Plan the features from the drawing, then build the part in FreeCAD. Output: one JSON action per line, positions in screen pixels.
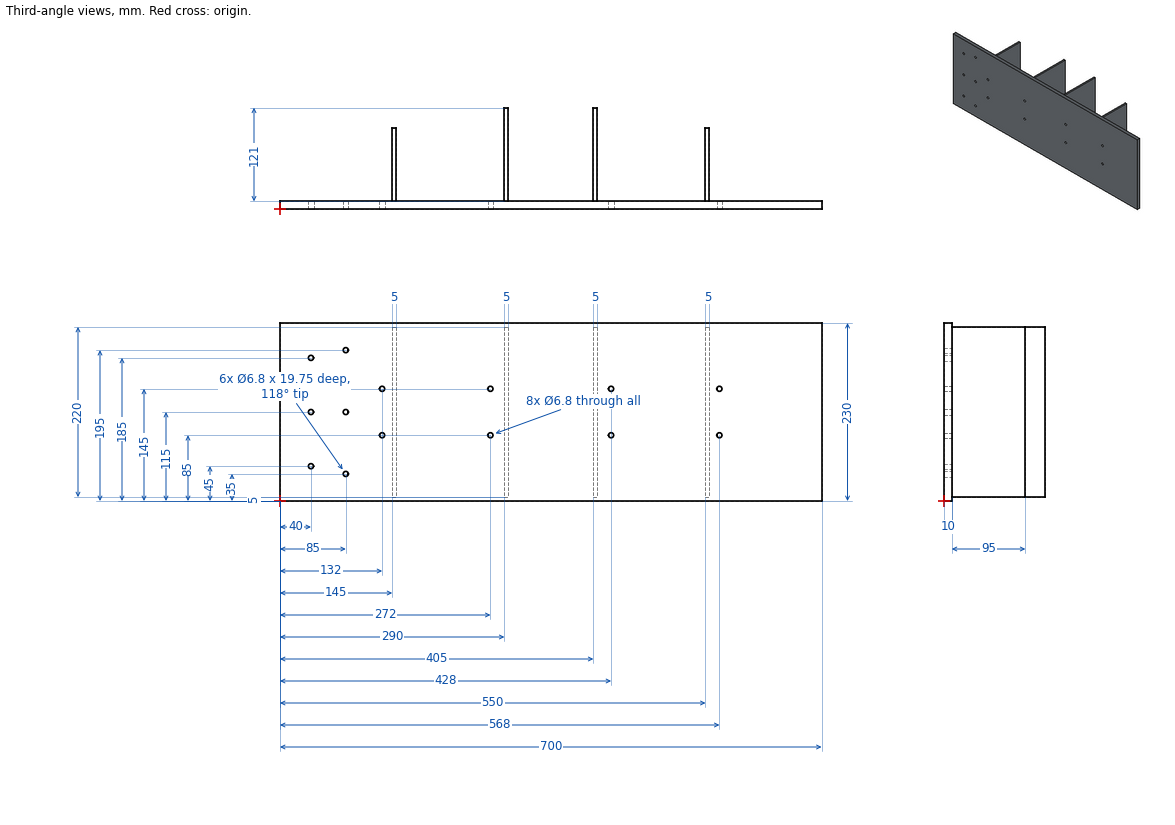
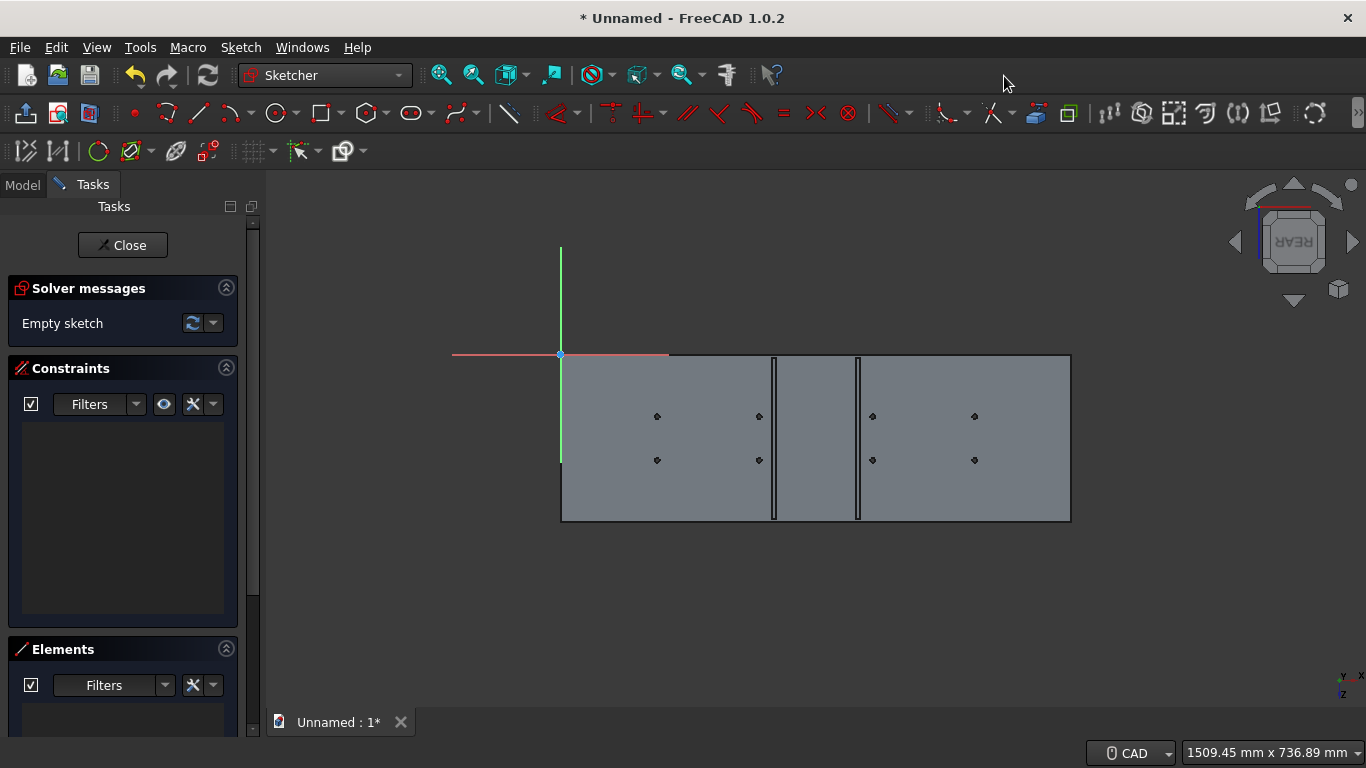
{"action": "scroll", "coordinate": [795, 433], "scroll_direction": "up", "scroll_amount": 2}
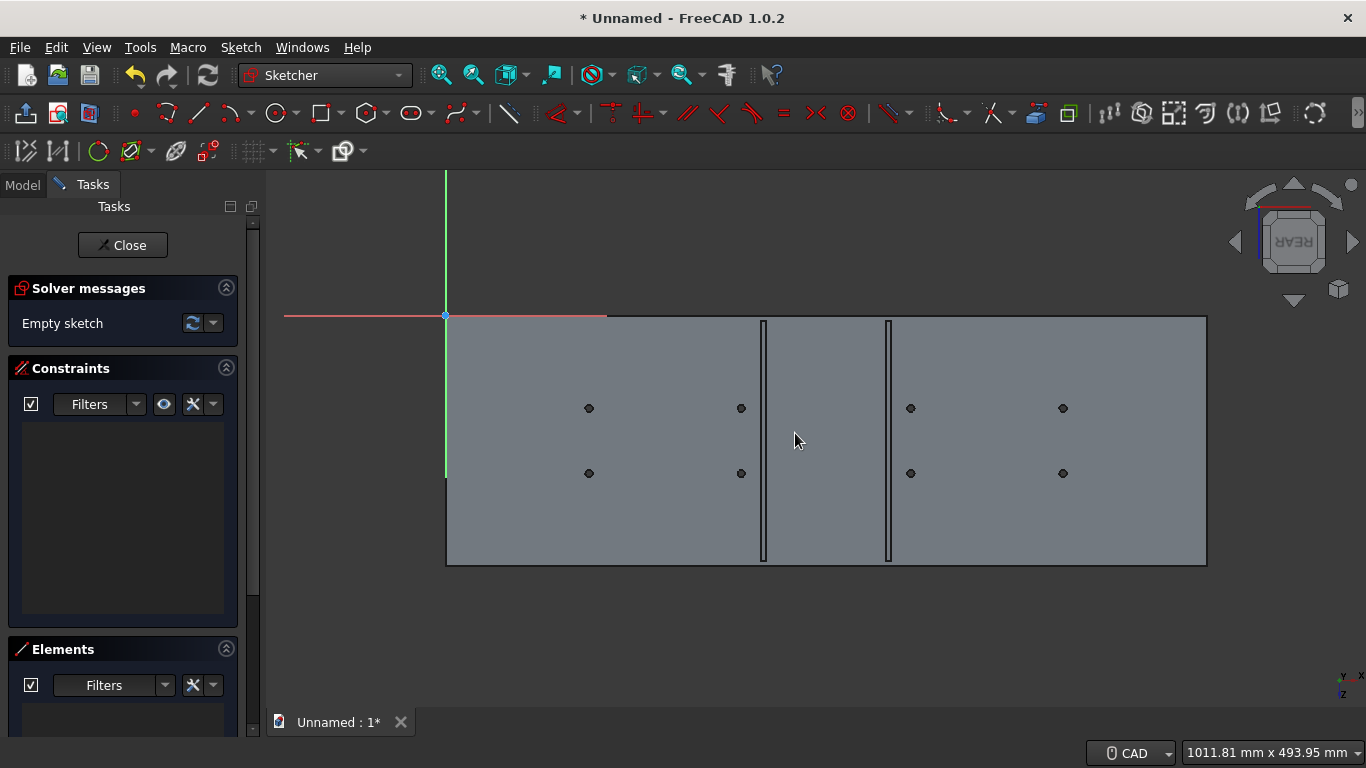
{"action": "key", "text": "g r"}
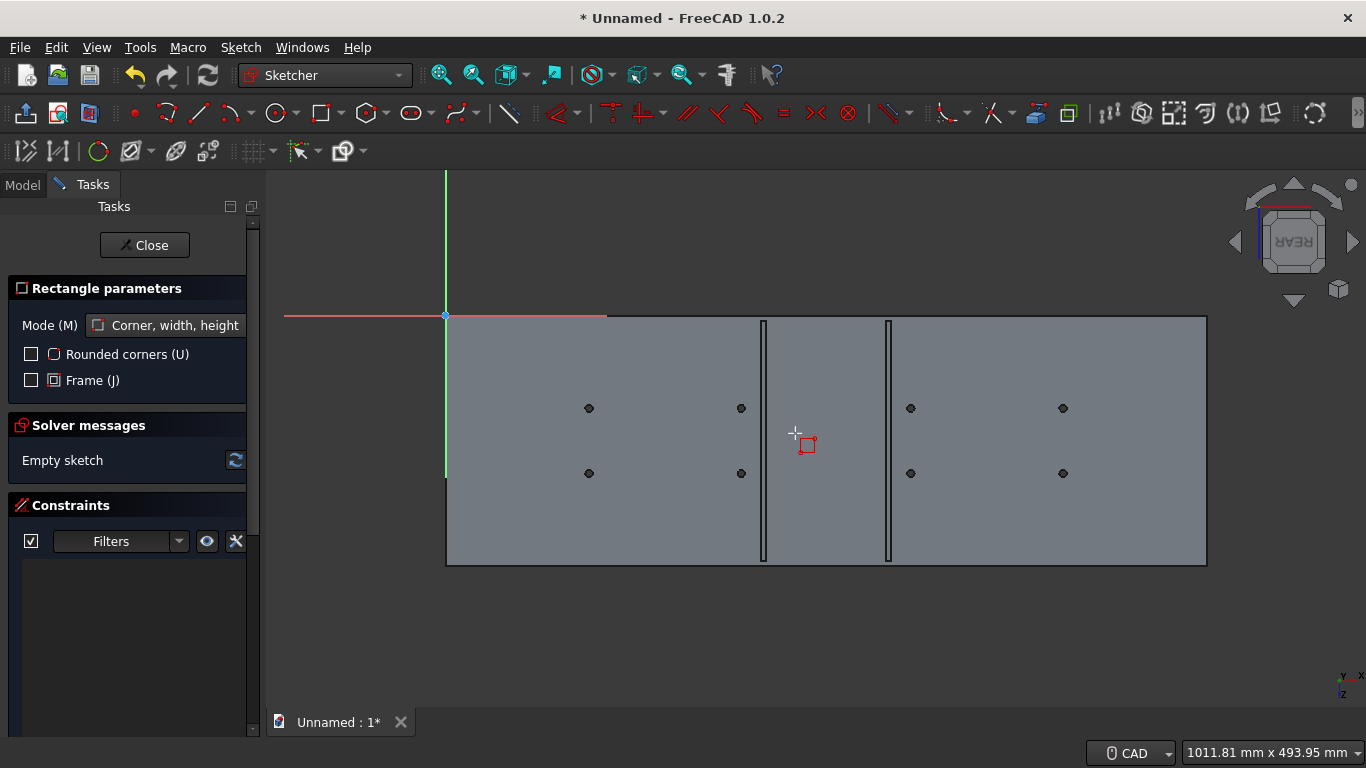
{"action": "scroll", "coordinate": [603, 321], "scroll_direction": "up", "scroll_amount": 6}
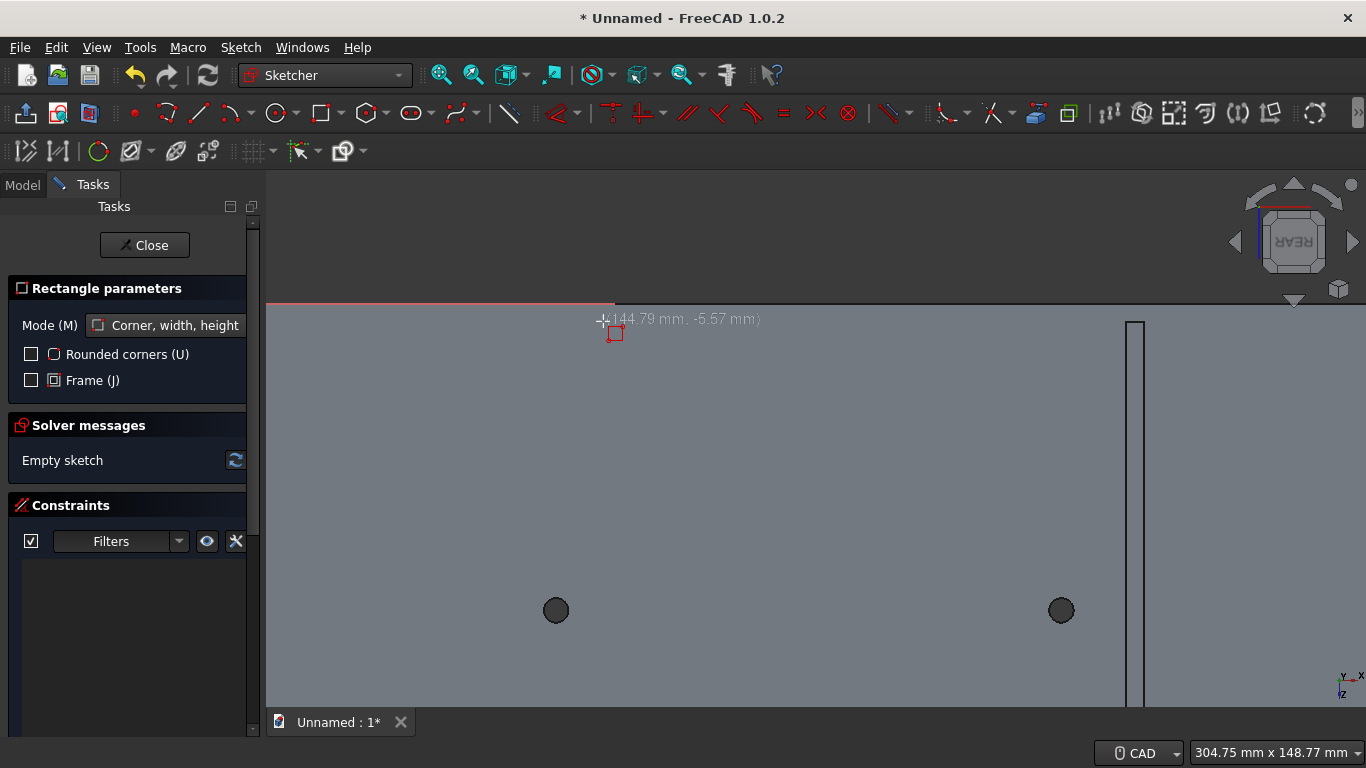
{"action": "left_click", "coordinate": [603, 322]}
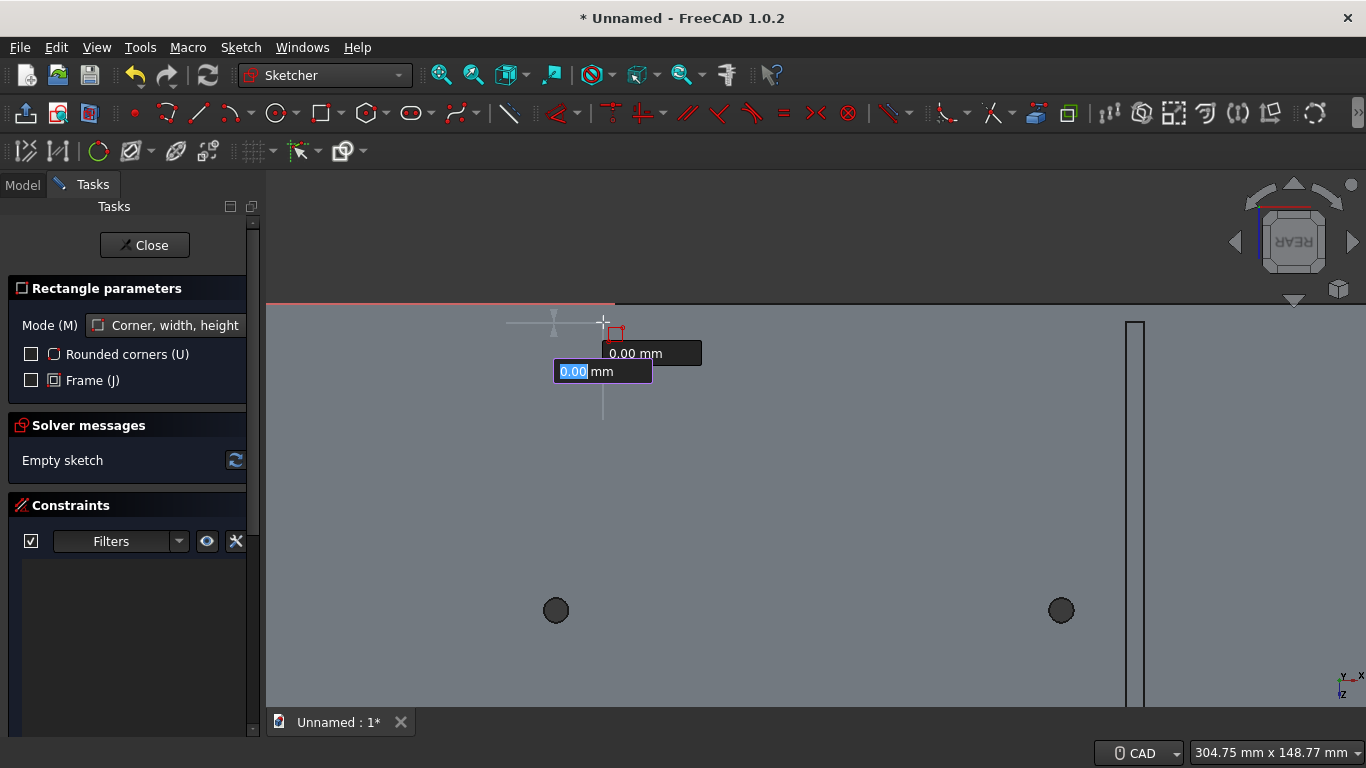
{"action": "scroll", "coordinate": [604, 322], "scroll_direction": "down", "scroll_amount": 6}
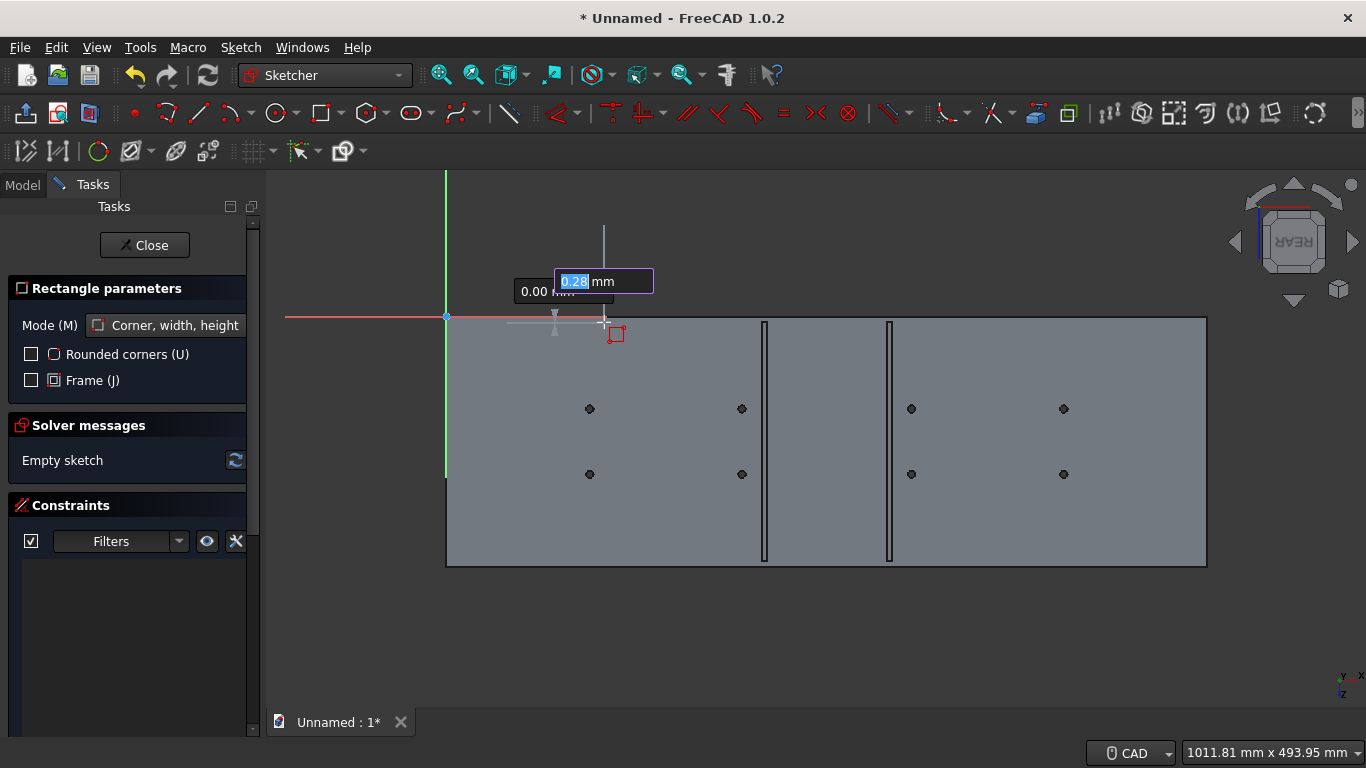
{"action": "left_click", "coordinate": [609, 561]}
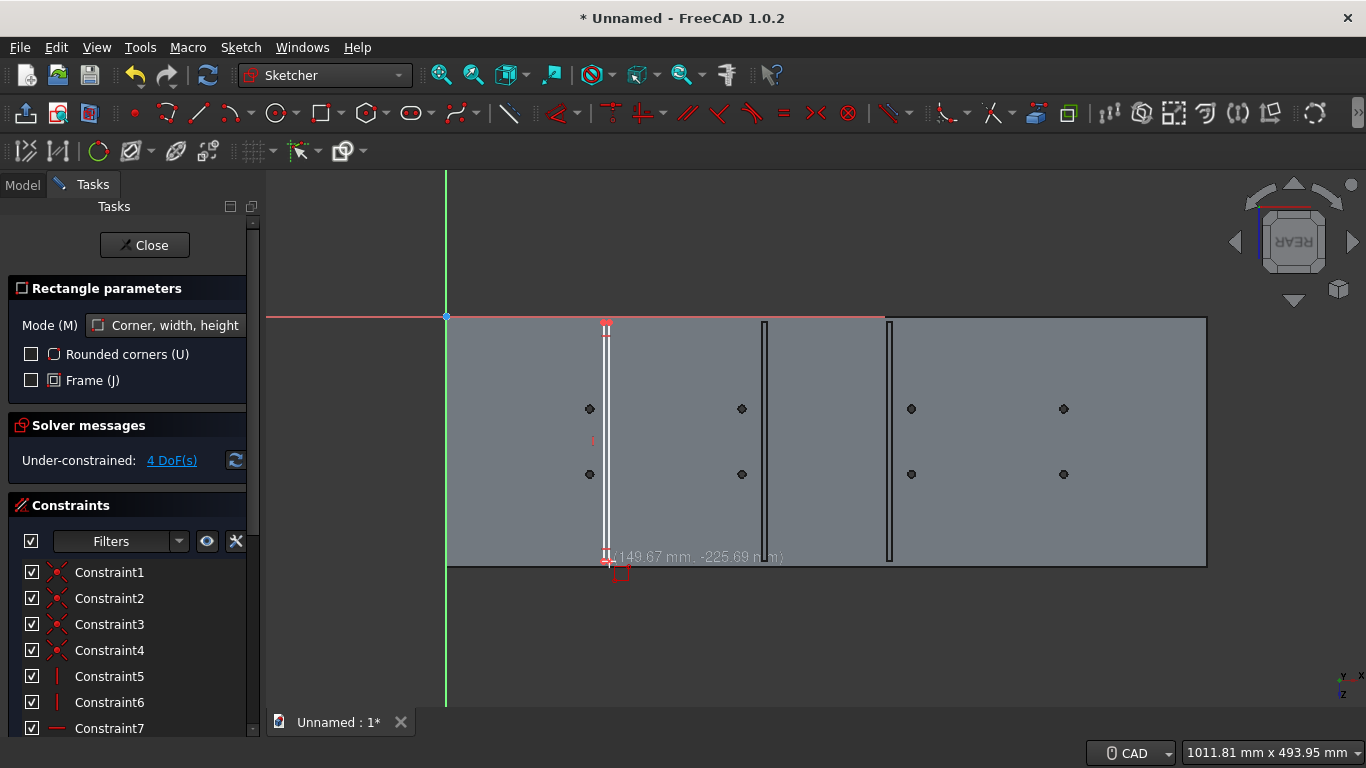
{"action": "scroll", "coordinate": [1044, 322], "scroll_direction": "up", "scroll_amount": 6}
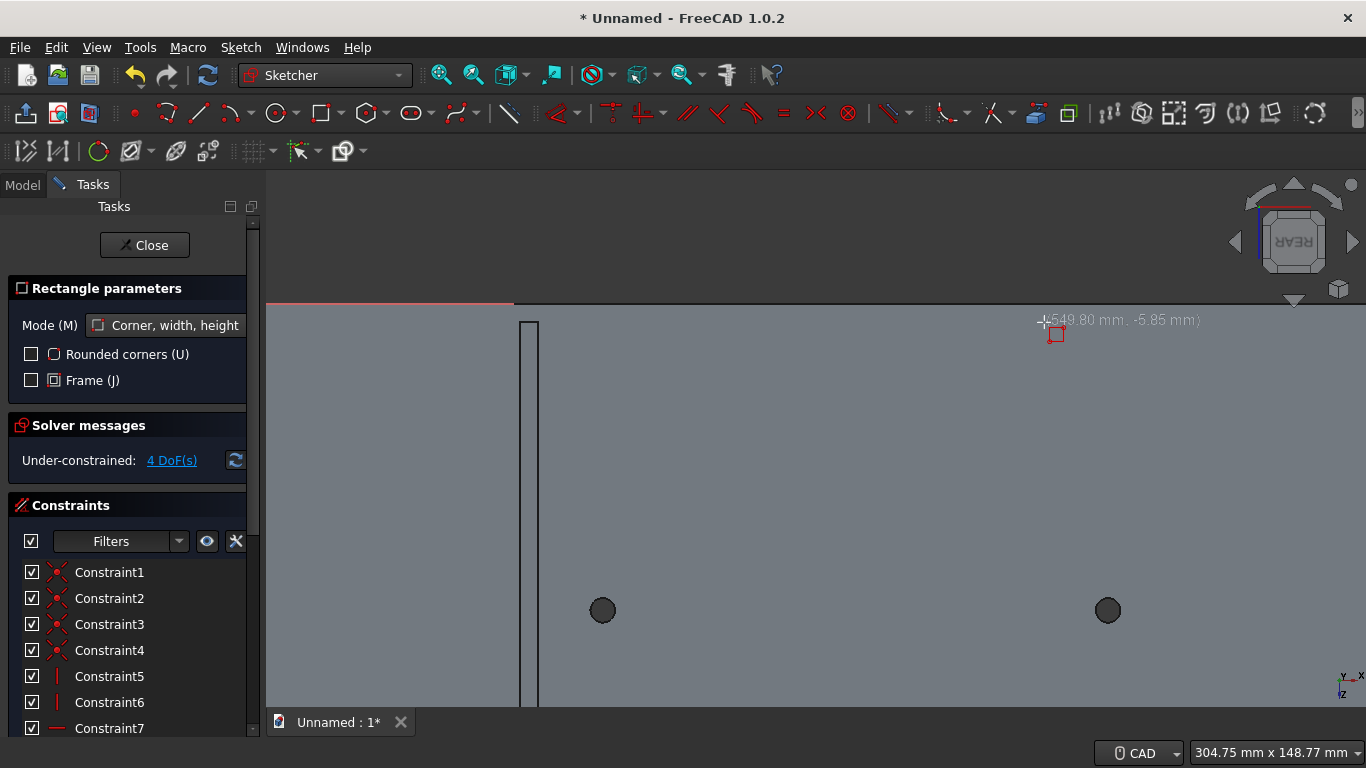
{"action": "left_click", "coordinate": [1043, 322]}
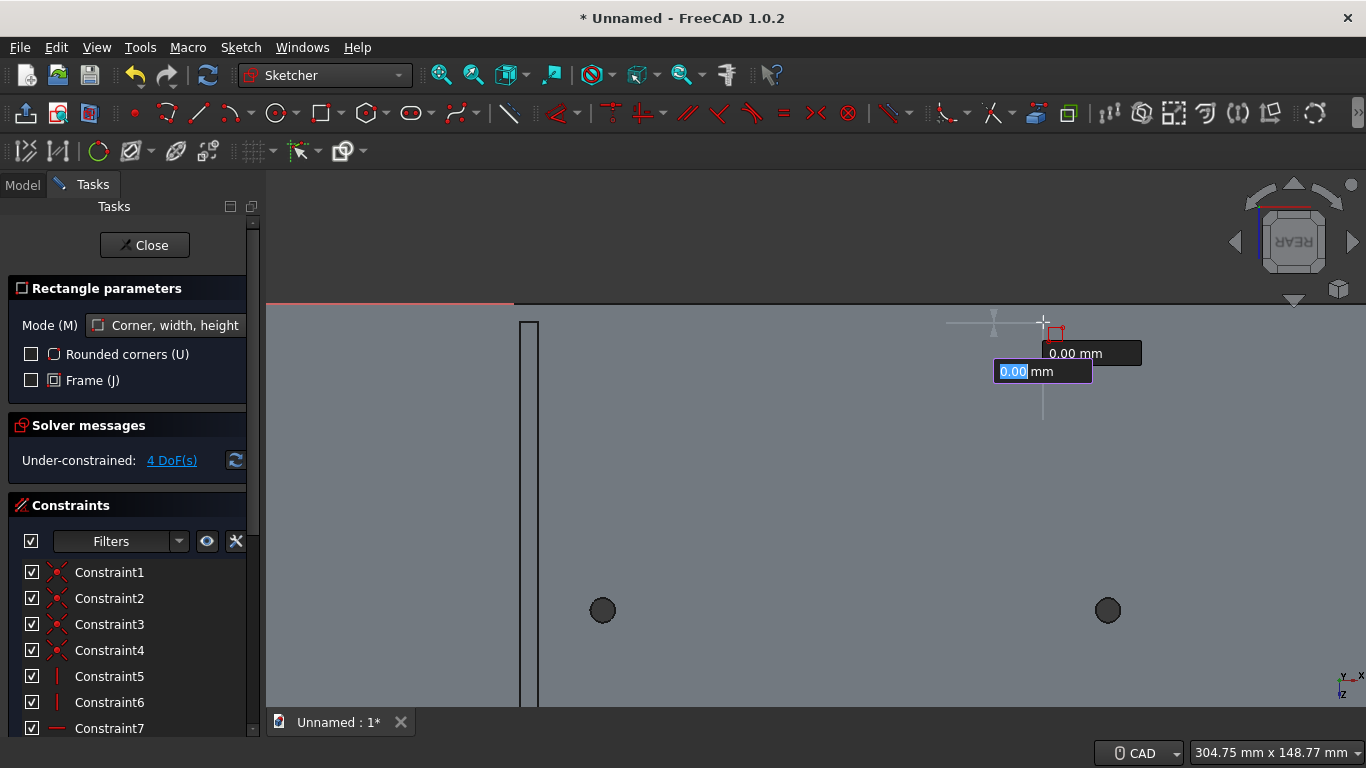
{"action": "scroll", "coordinate": [1044, 322], "scroll_direction": "down", "scroll_amount": 6}